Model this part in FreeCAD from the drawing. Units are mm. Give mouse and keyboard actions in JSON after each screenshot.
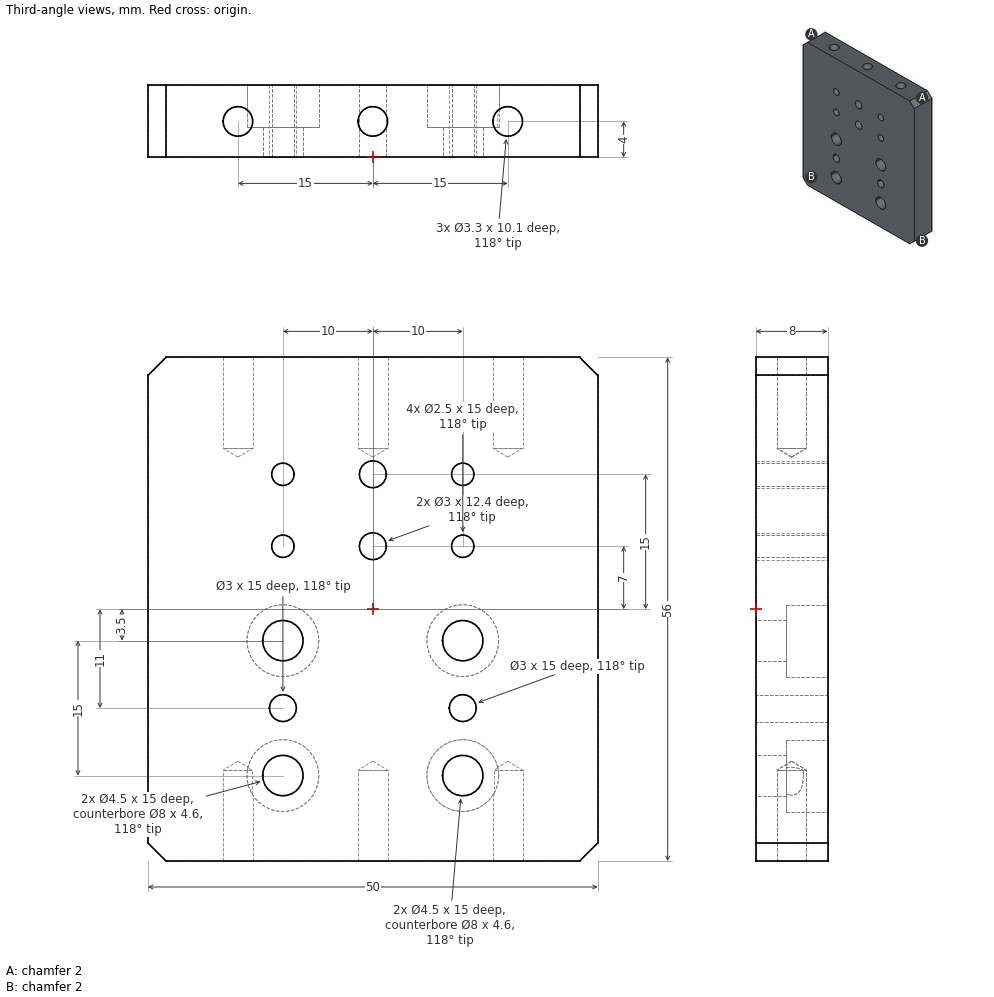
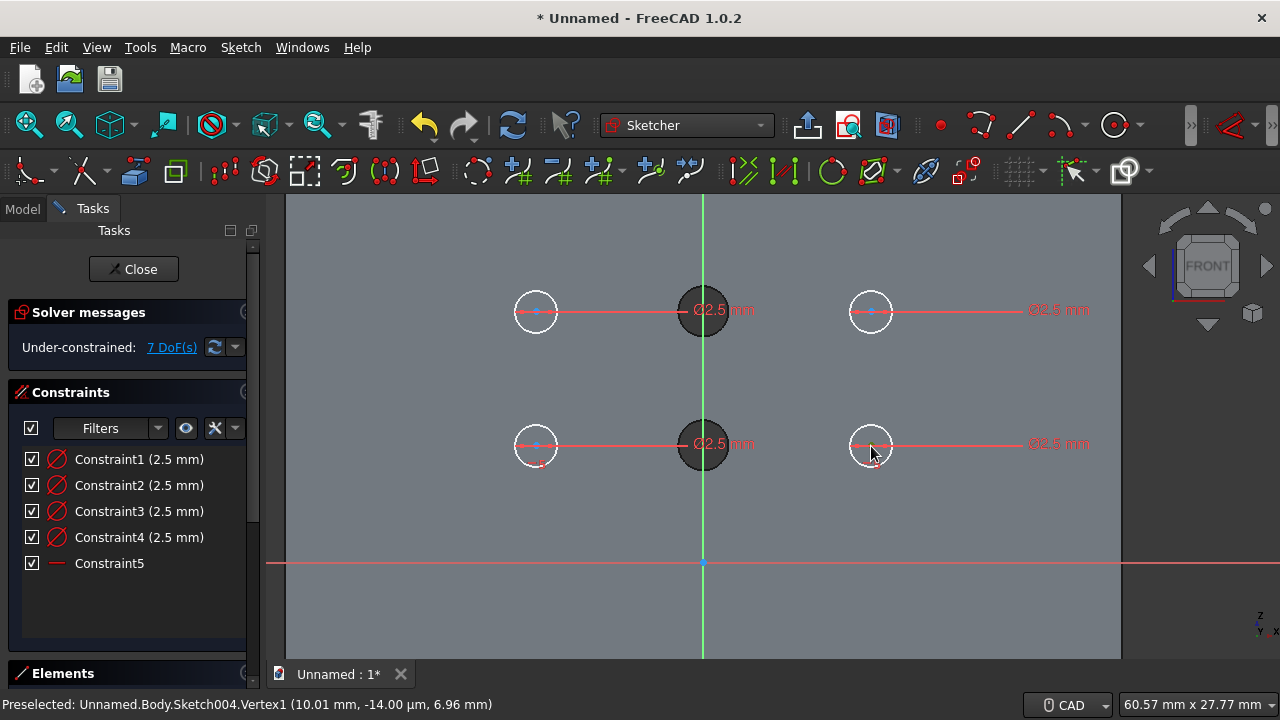
{"action": "left_click", "coordinate": [871, 312]}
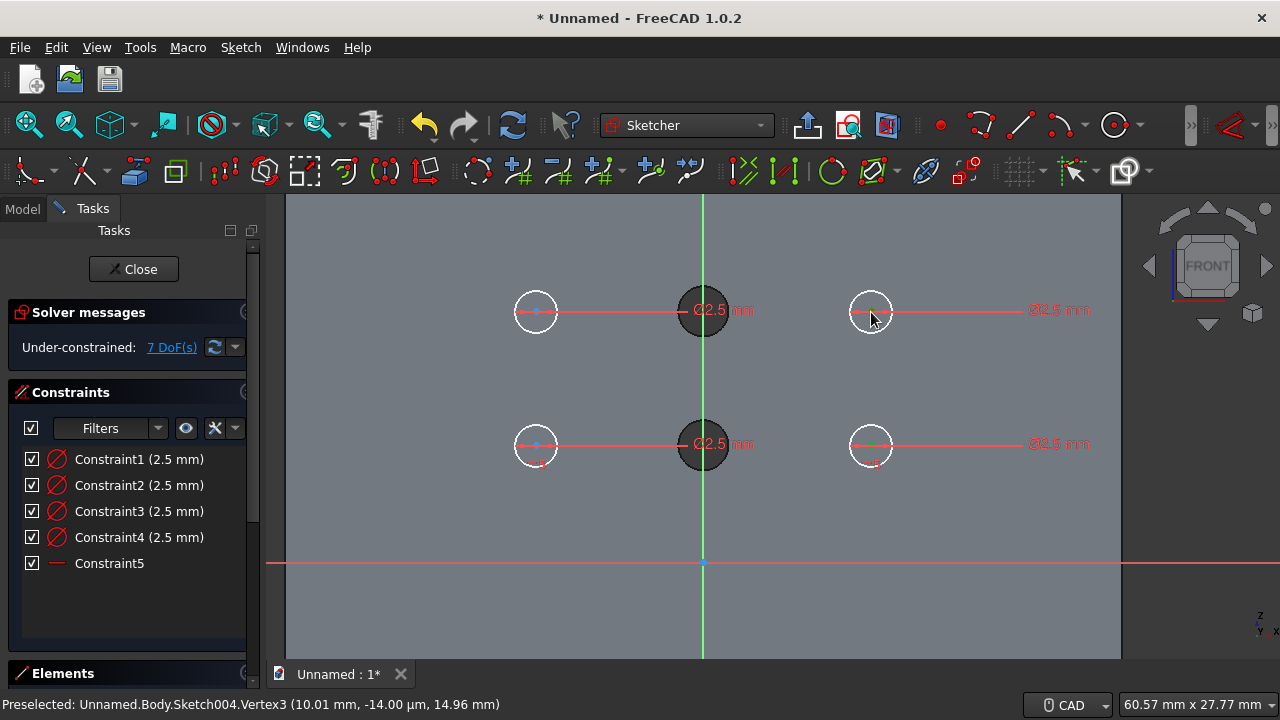
{"action": "key", "text": "v"}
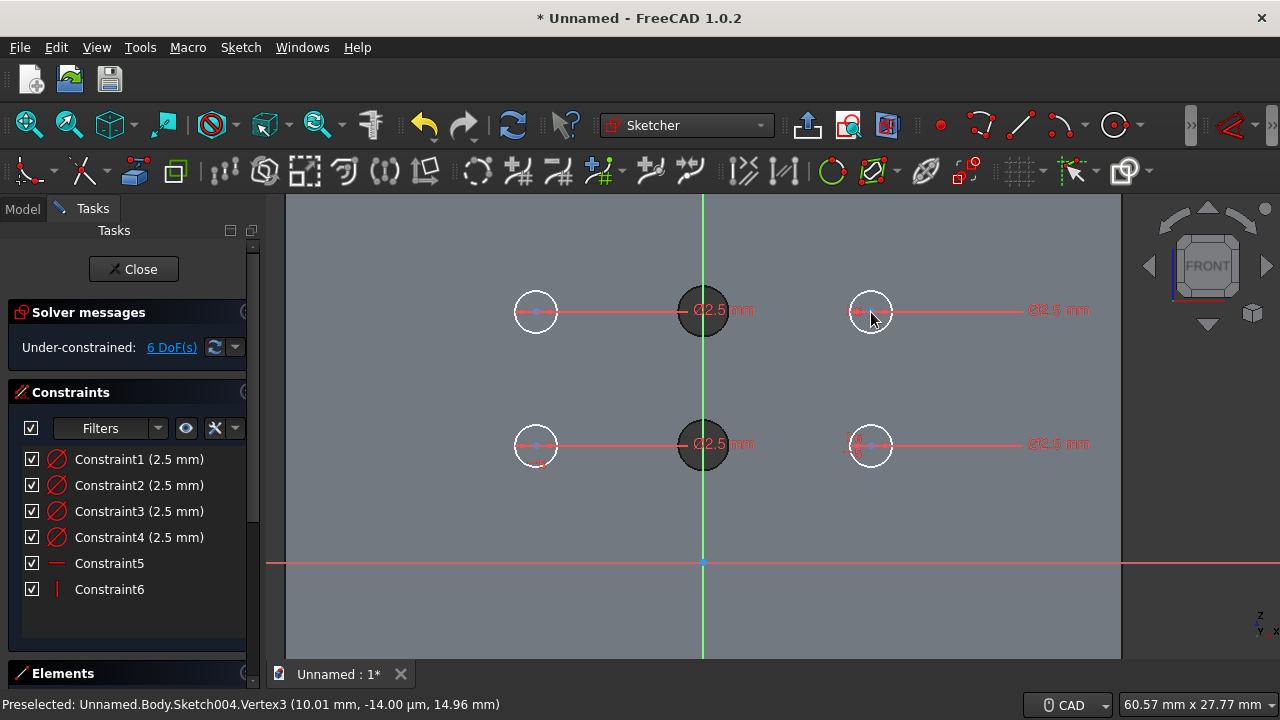
{"action": "left_click", "coordinate": [536, 446]}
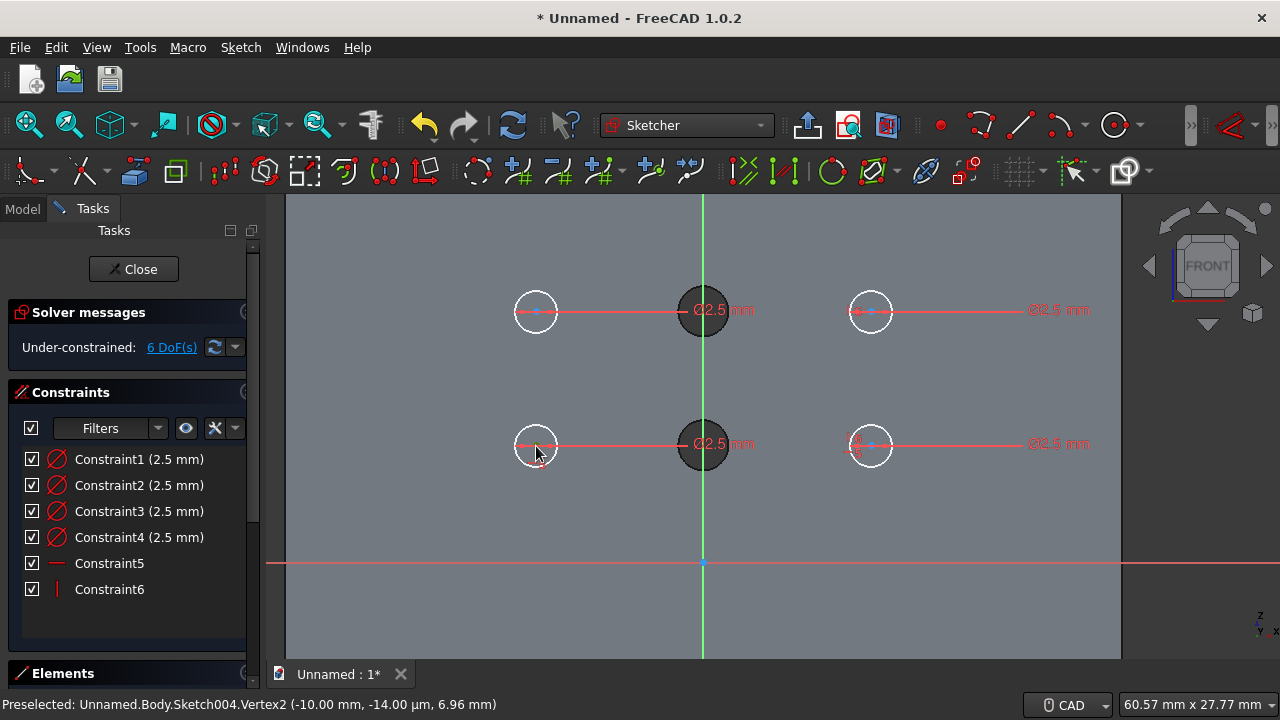
{"action": "left_click", "coordinate": [536, 312]}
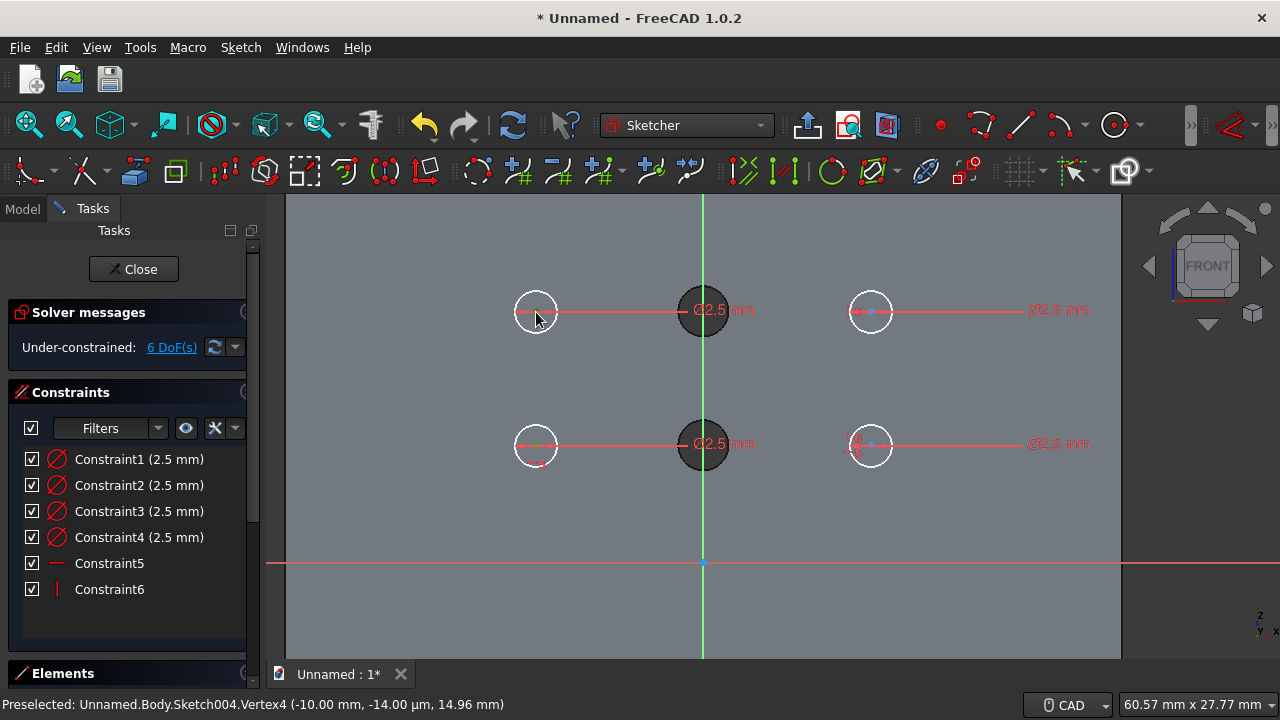
{"action": "key", "text": "v"}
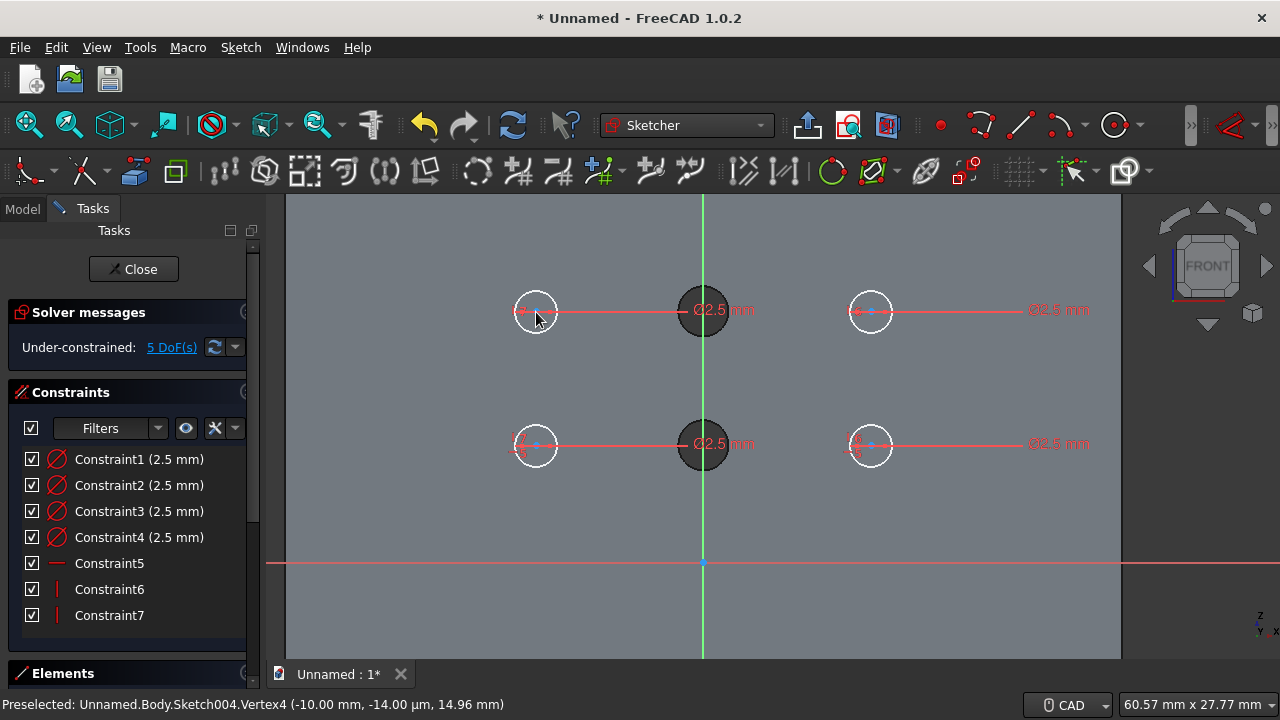
{"action": "left_click", "coordinate": [871, 312]}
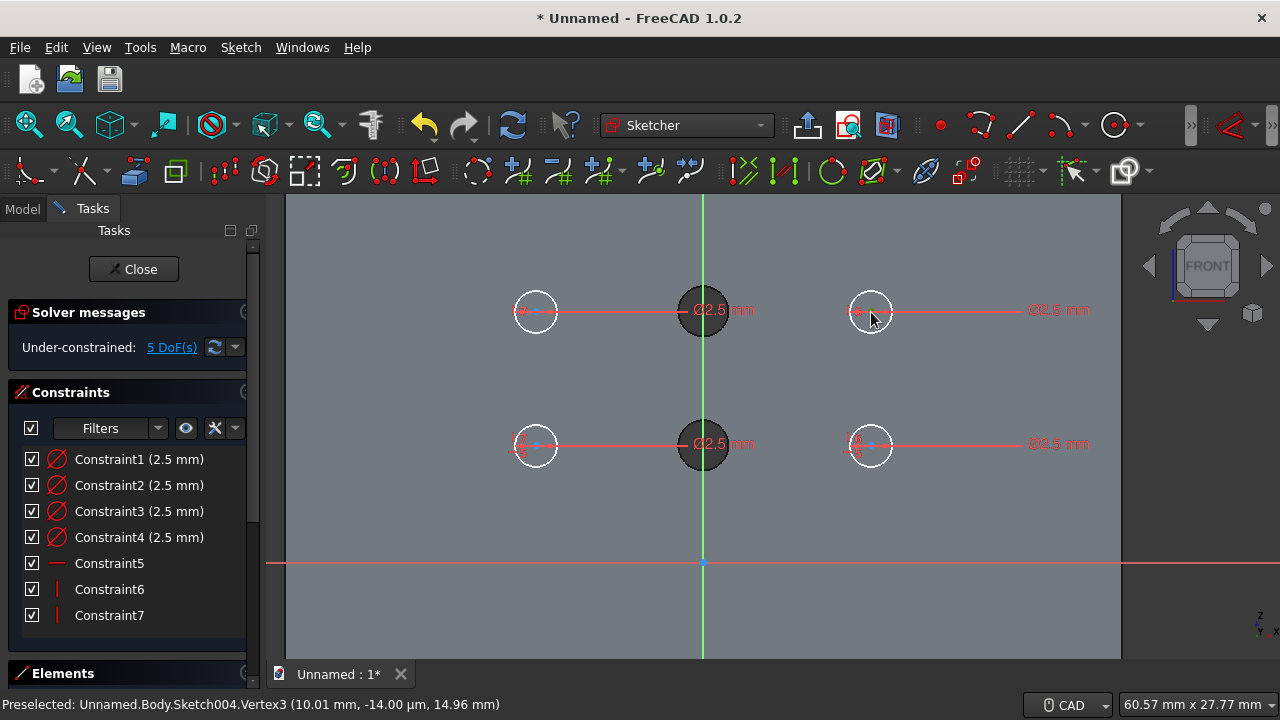
{"action": "left_click", "coordinate": [536, 312]}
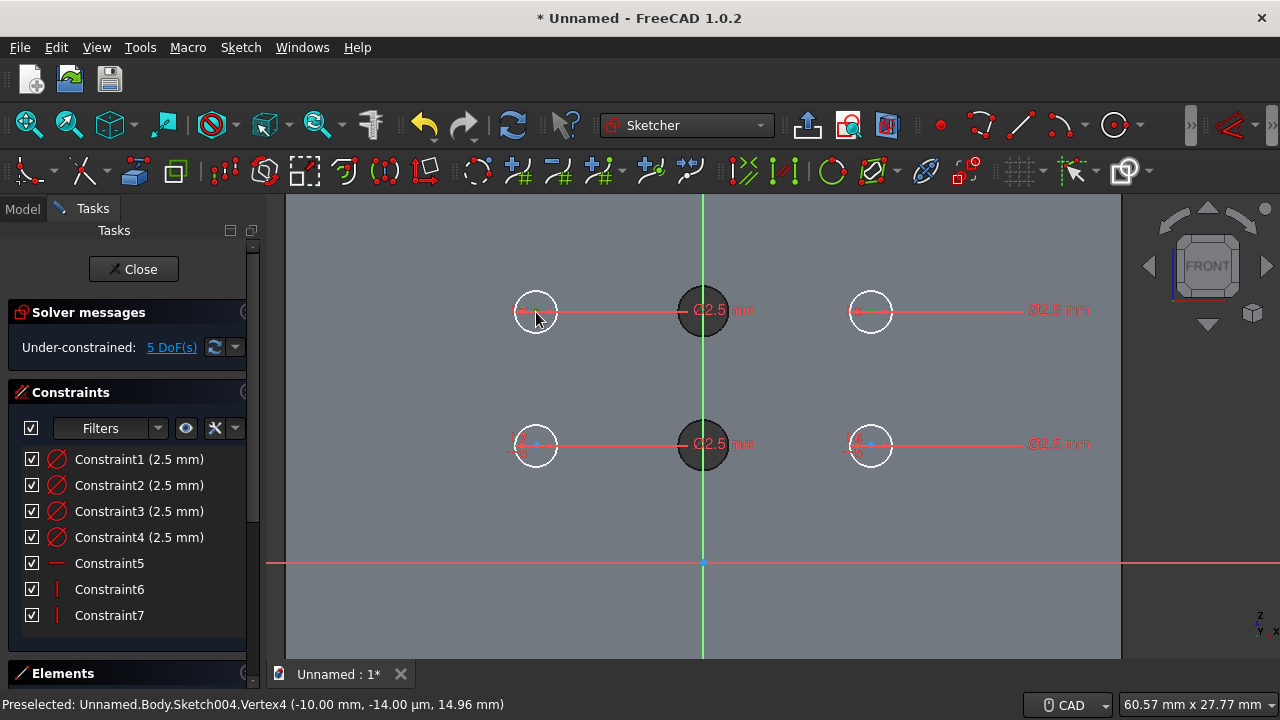
{"action": "key", "text": "h"}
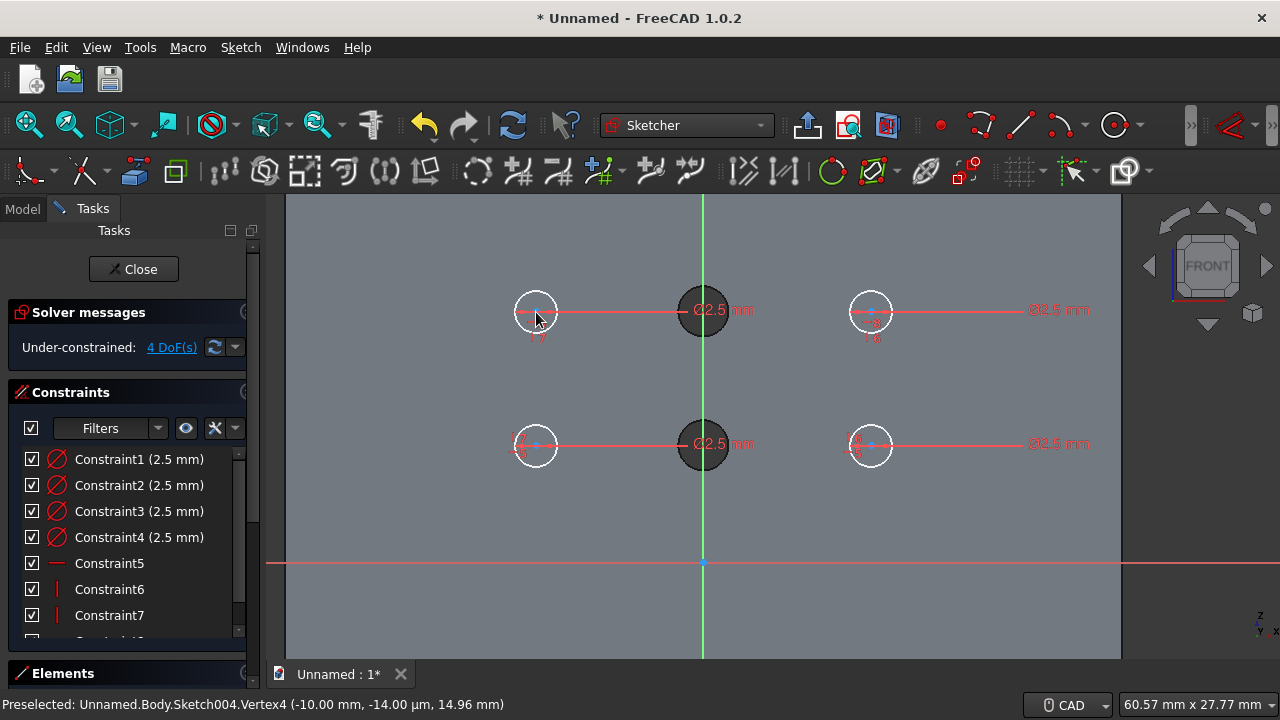
{"action": "left_click", "coordinate": [1230, 126]}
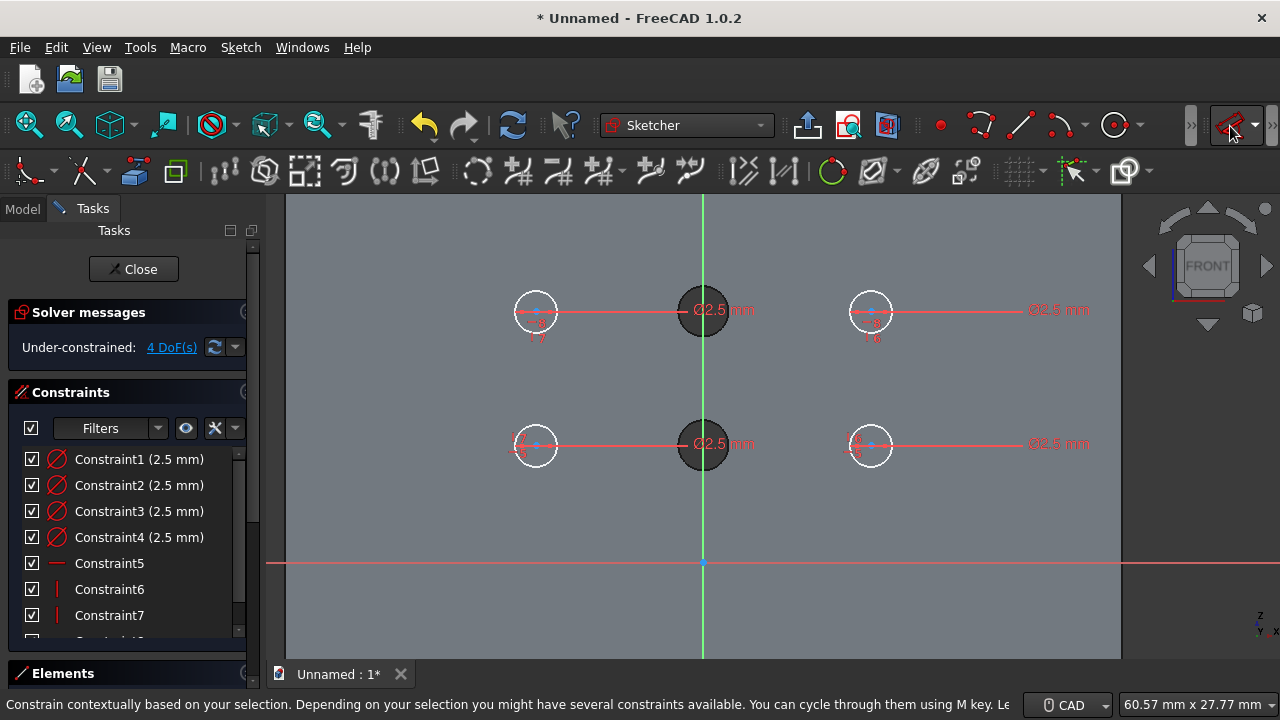
{"action": "left_click", "coordinate": [871, 446]}
{"action": "left_click", "coordinate": [905, 504]}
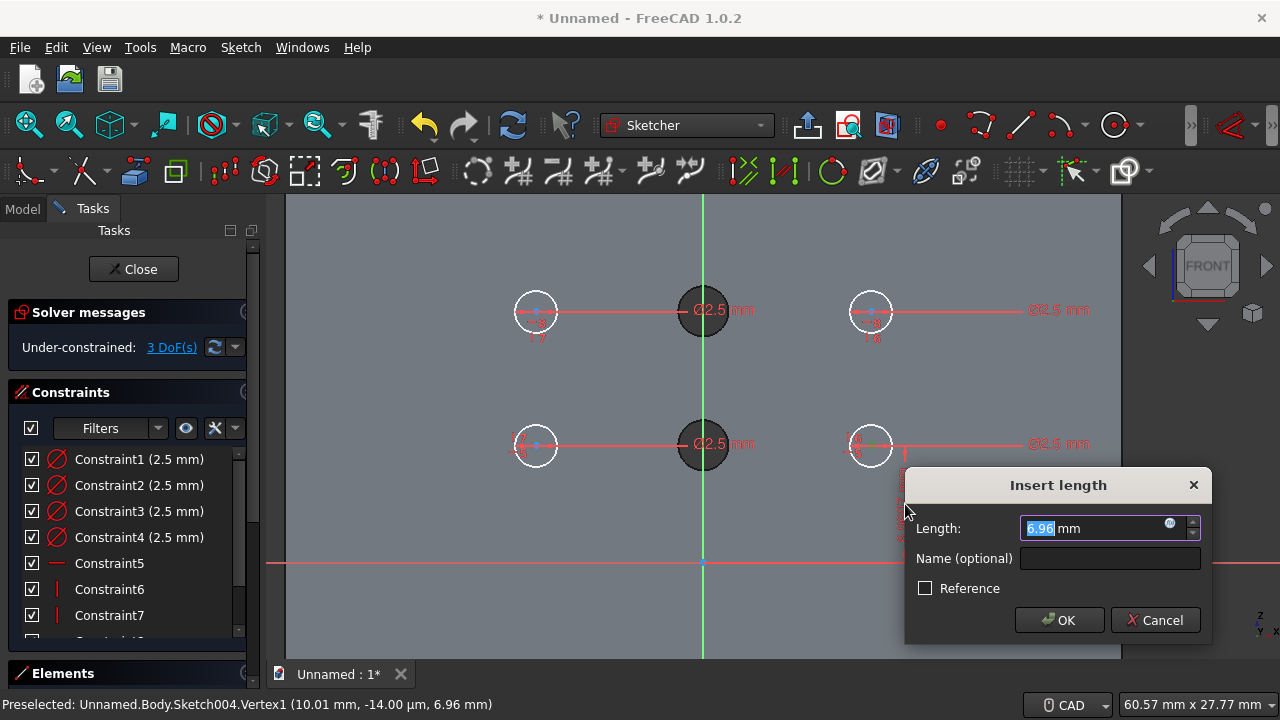
{"action": "type", "text": "7"}
{"action": "key", "text": "Return"}